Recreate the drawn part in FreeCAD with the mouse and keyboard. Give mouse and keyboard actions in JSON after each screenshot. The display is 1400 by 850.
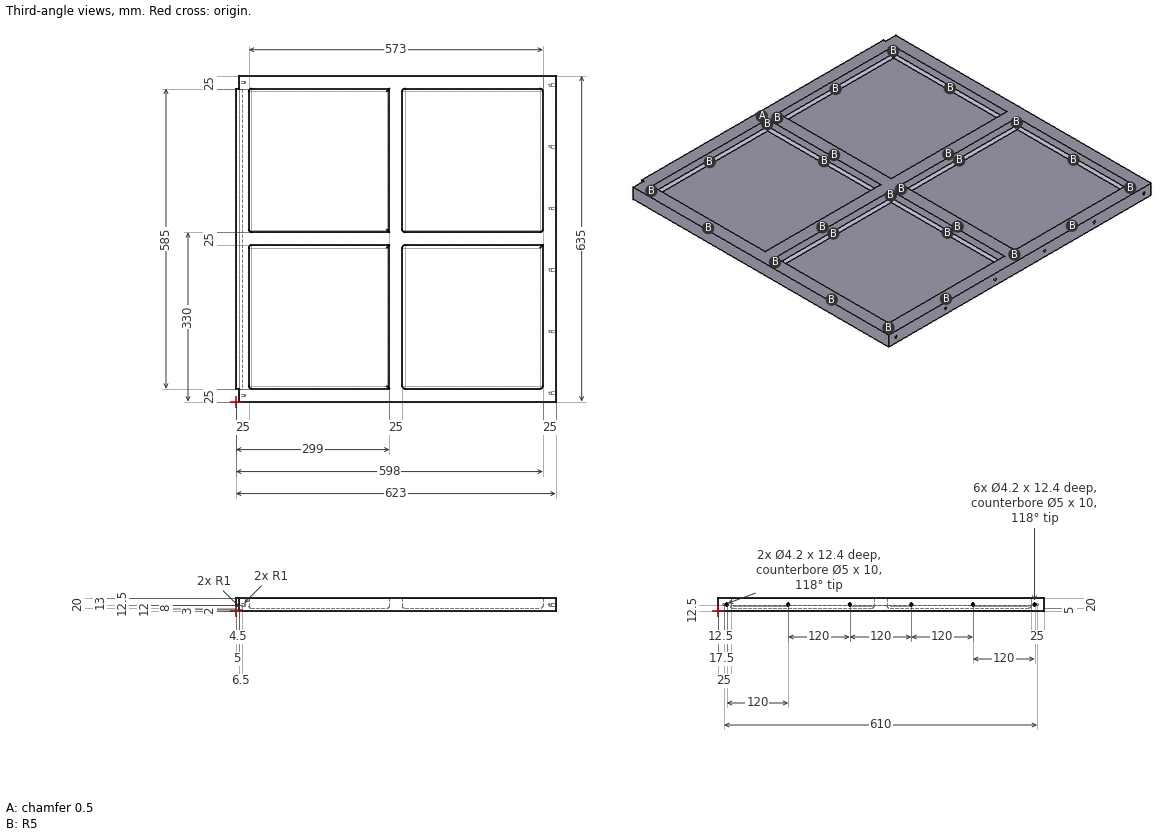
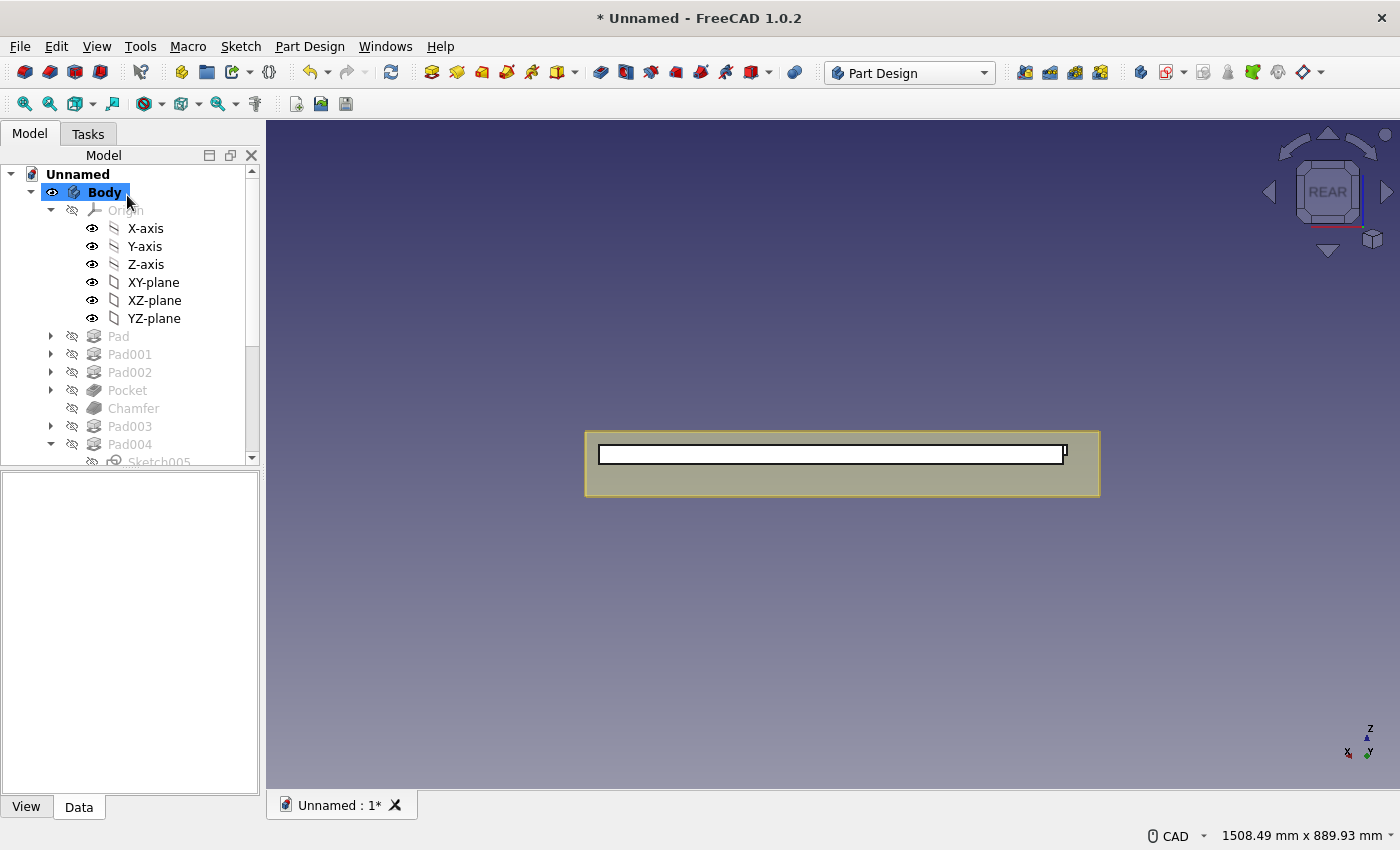
{"action": "scroll", "coordinate": [101, 314], "scroll_direction": "down", "scroll_amount": 3}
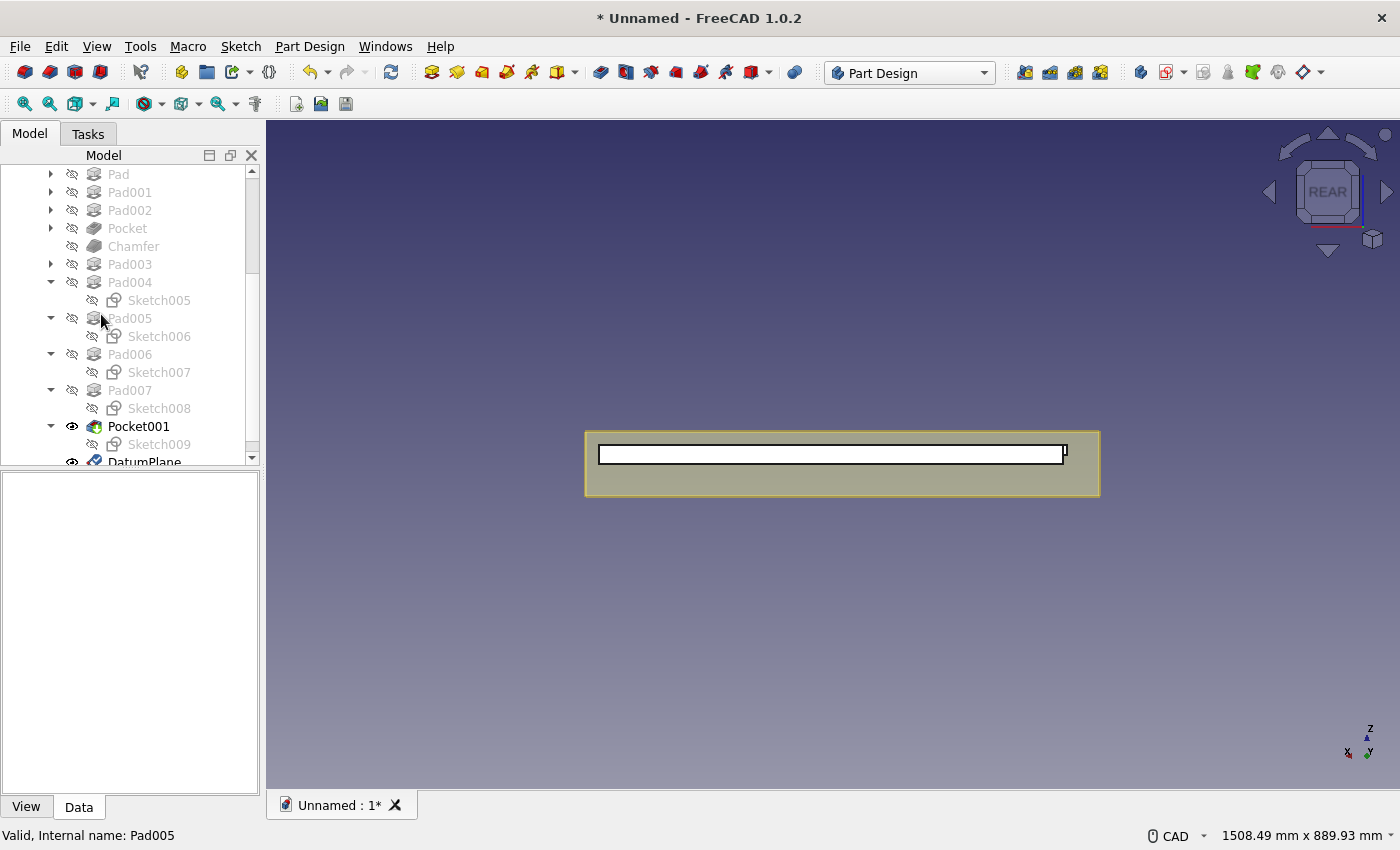
{"action": "left_click", "coordinate": [117, 462]}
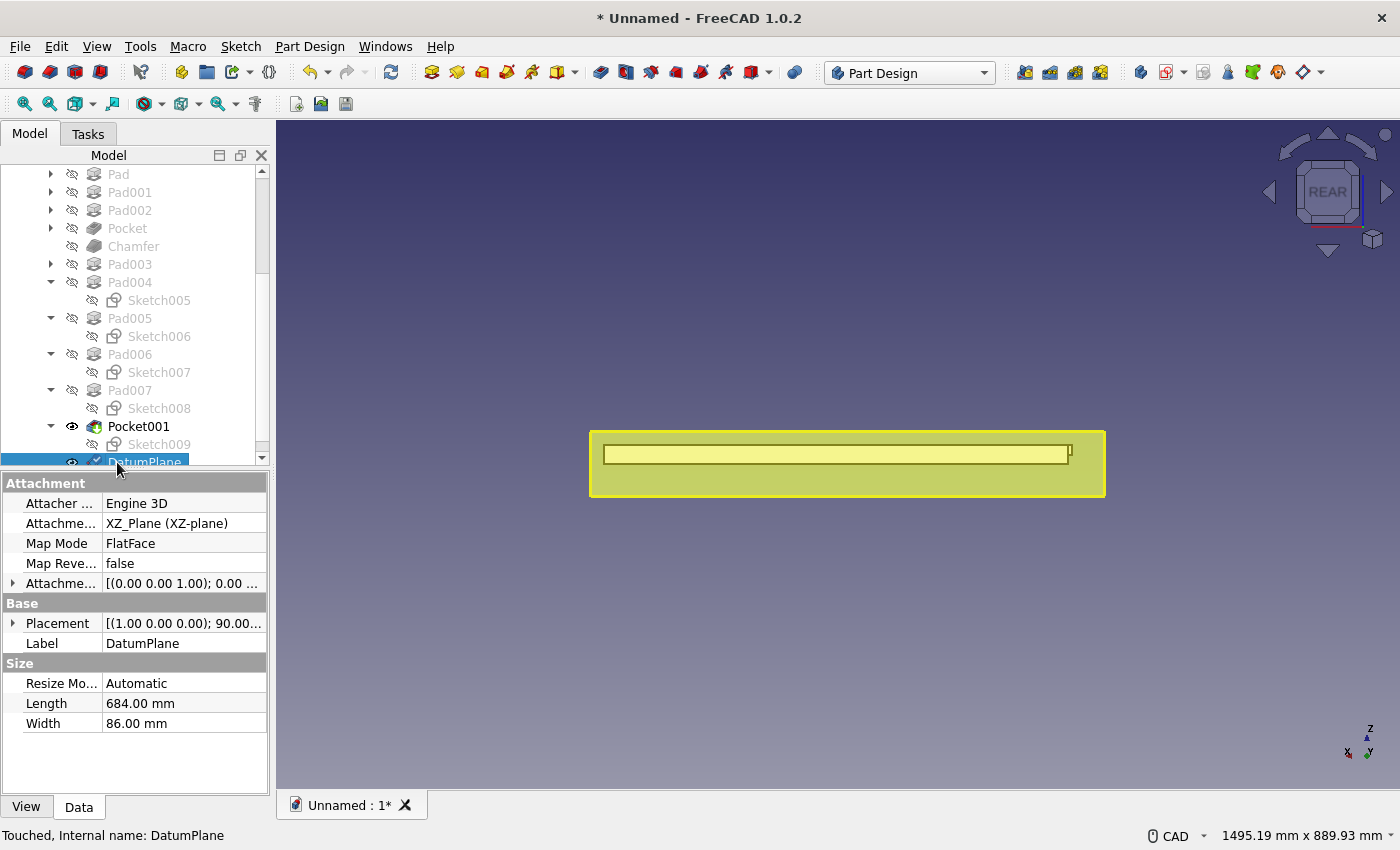
{"action": "left_click", "coordinate": [1166, 72]}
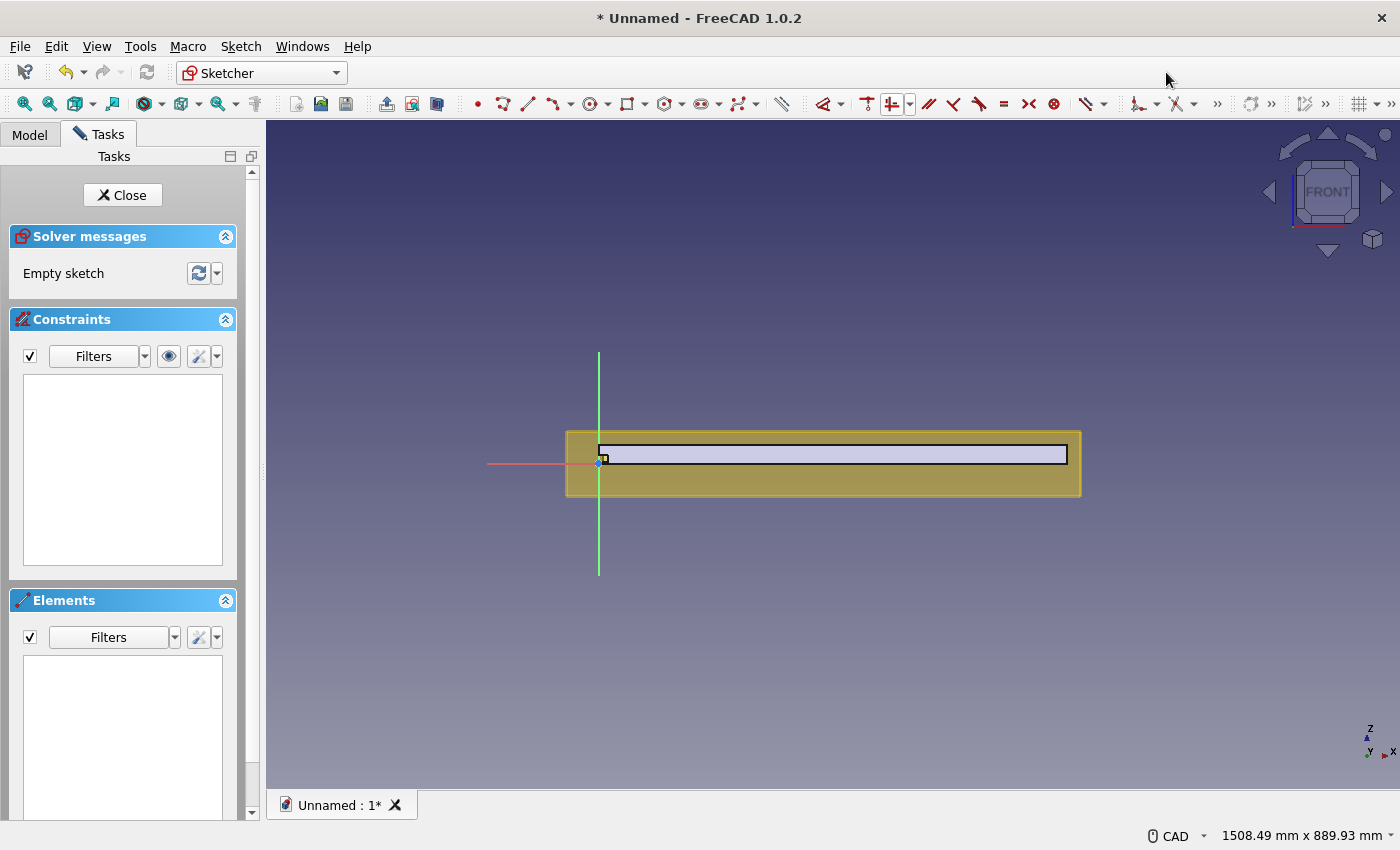
{"action": "left_click", "coordinate": [437, 104]}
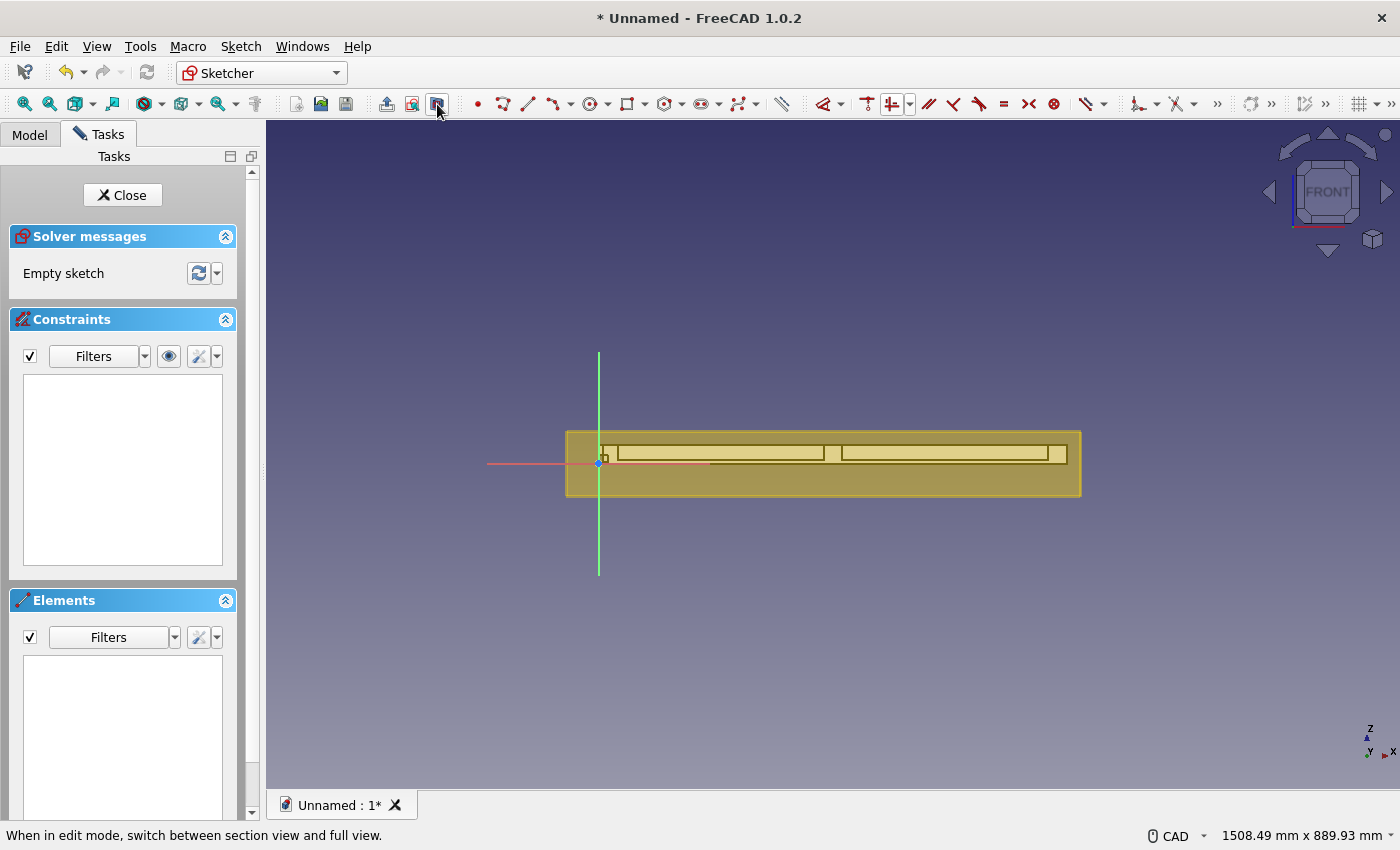
{"action": "scroll", "coordinate": [595, 460], "scroll_direction": "up", "scroll_amount": 15}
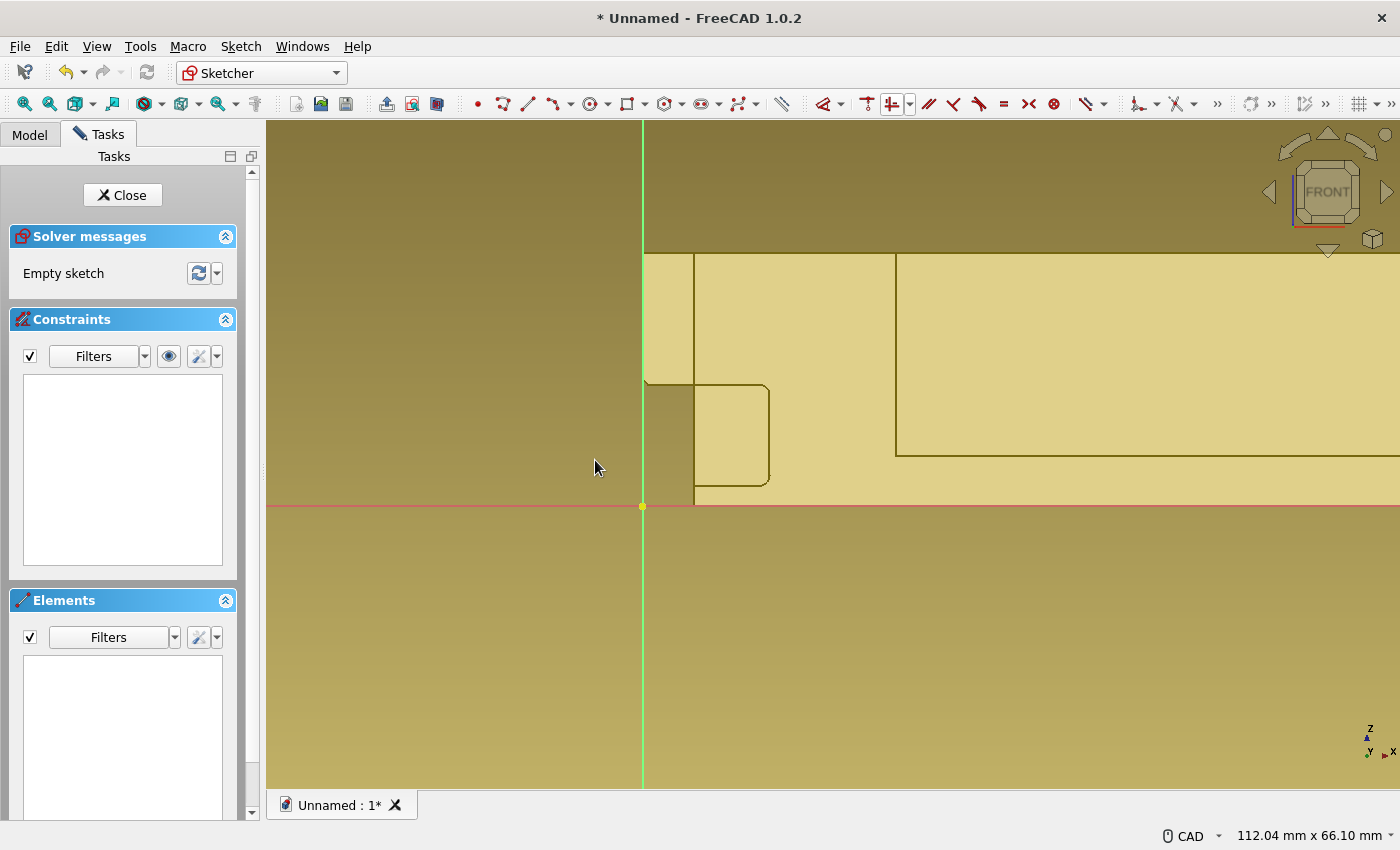
{"action": "scroll", "coordinate": [758, 424], "scroll_direction": "up", "scroll_amount": 4}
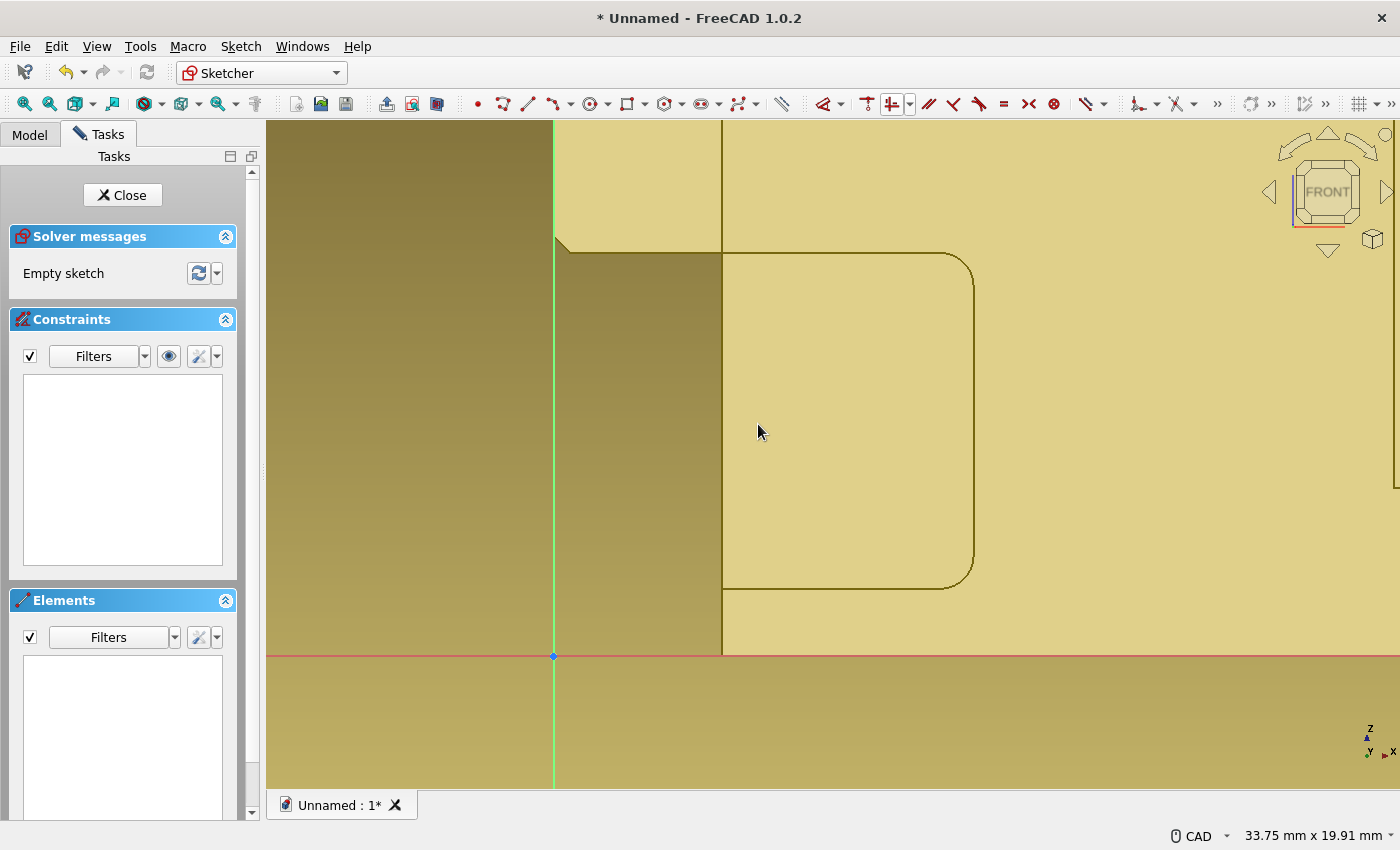
{"action": "left_click", "coordinate": [528, 104]}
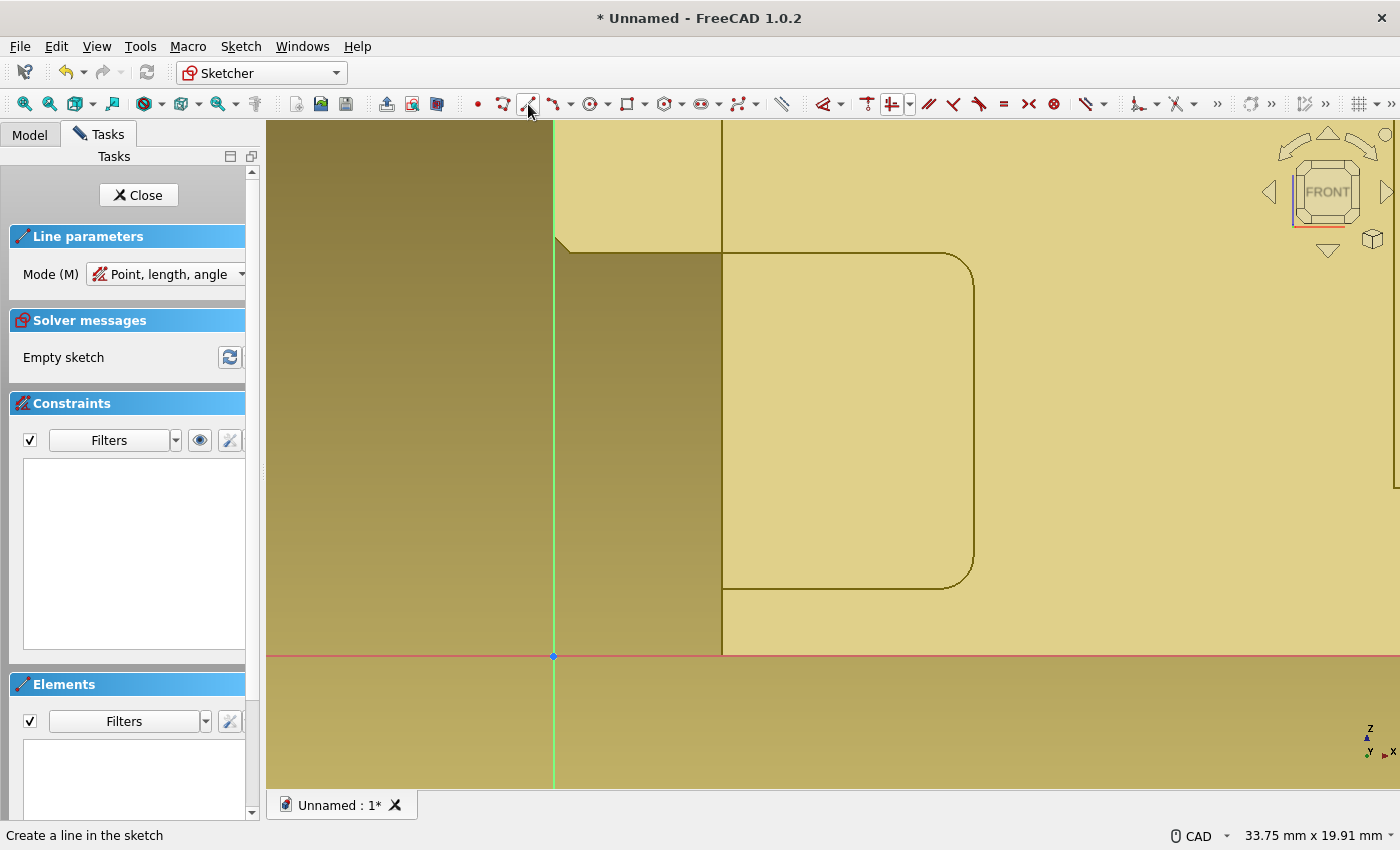
{"action": "left_click", "coordinate": [974, 555]}
{"action": "left_click", "coordinate": [974, 286]}